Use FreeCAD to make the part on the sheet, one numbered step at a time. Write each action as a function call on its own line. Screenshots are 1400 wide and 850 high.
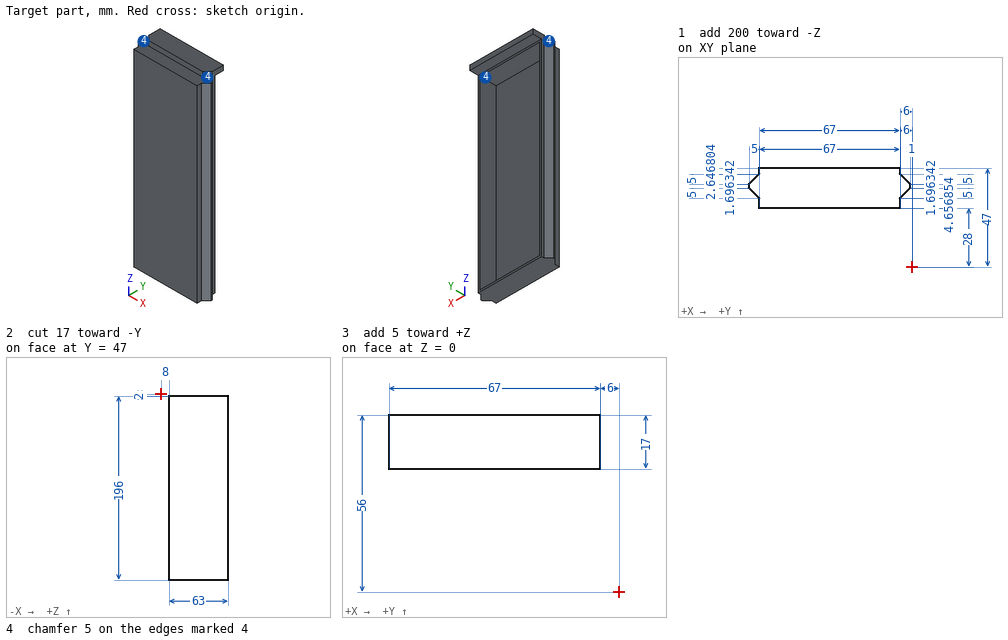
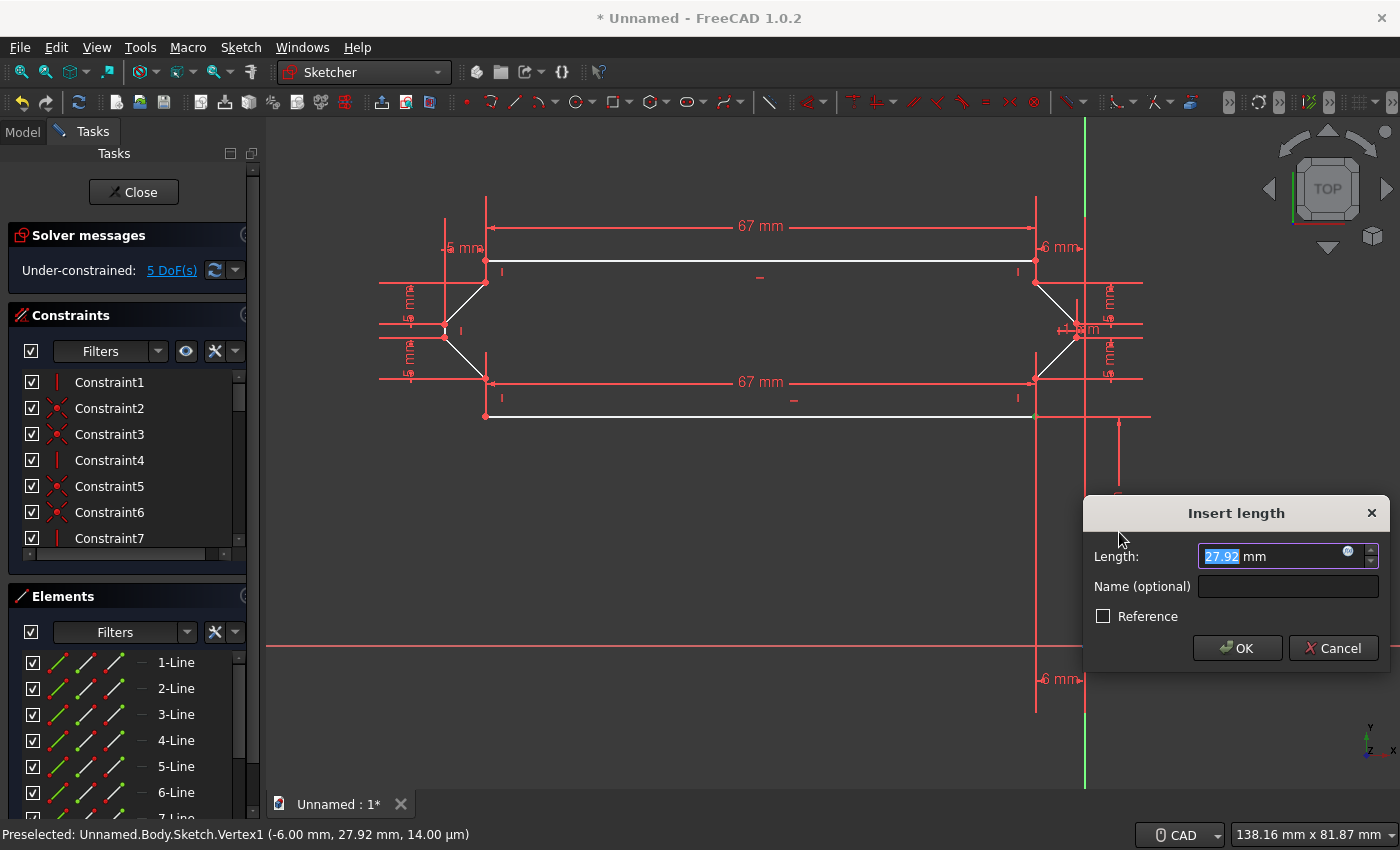
text(28)
key(Return)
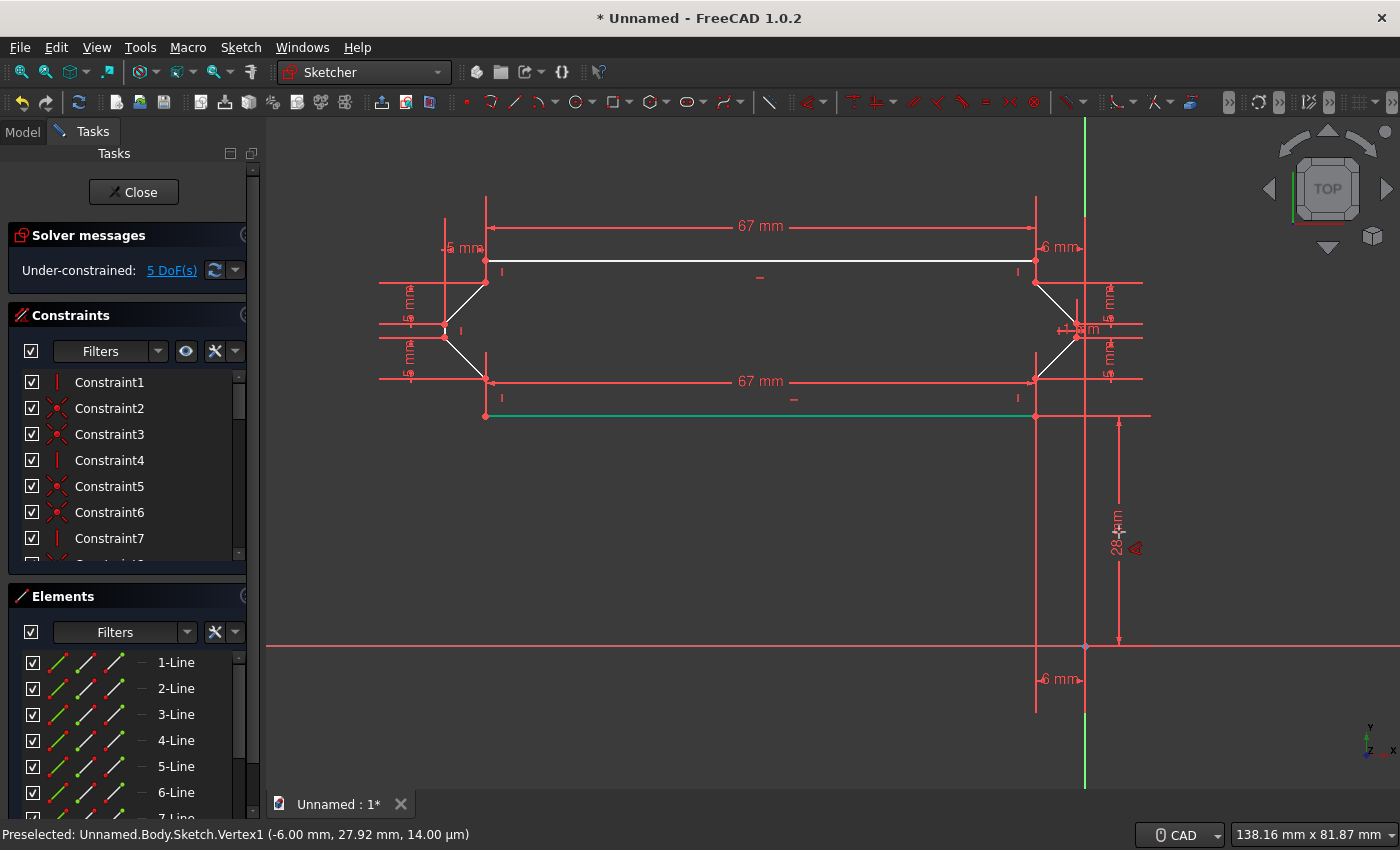
click(1036, 261)
click(1119, 454)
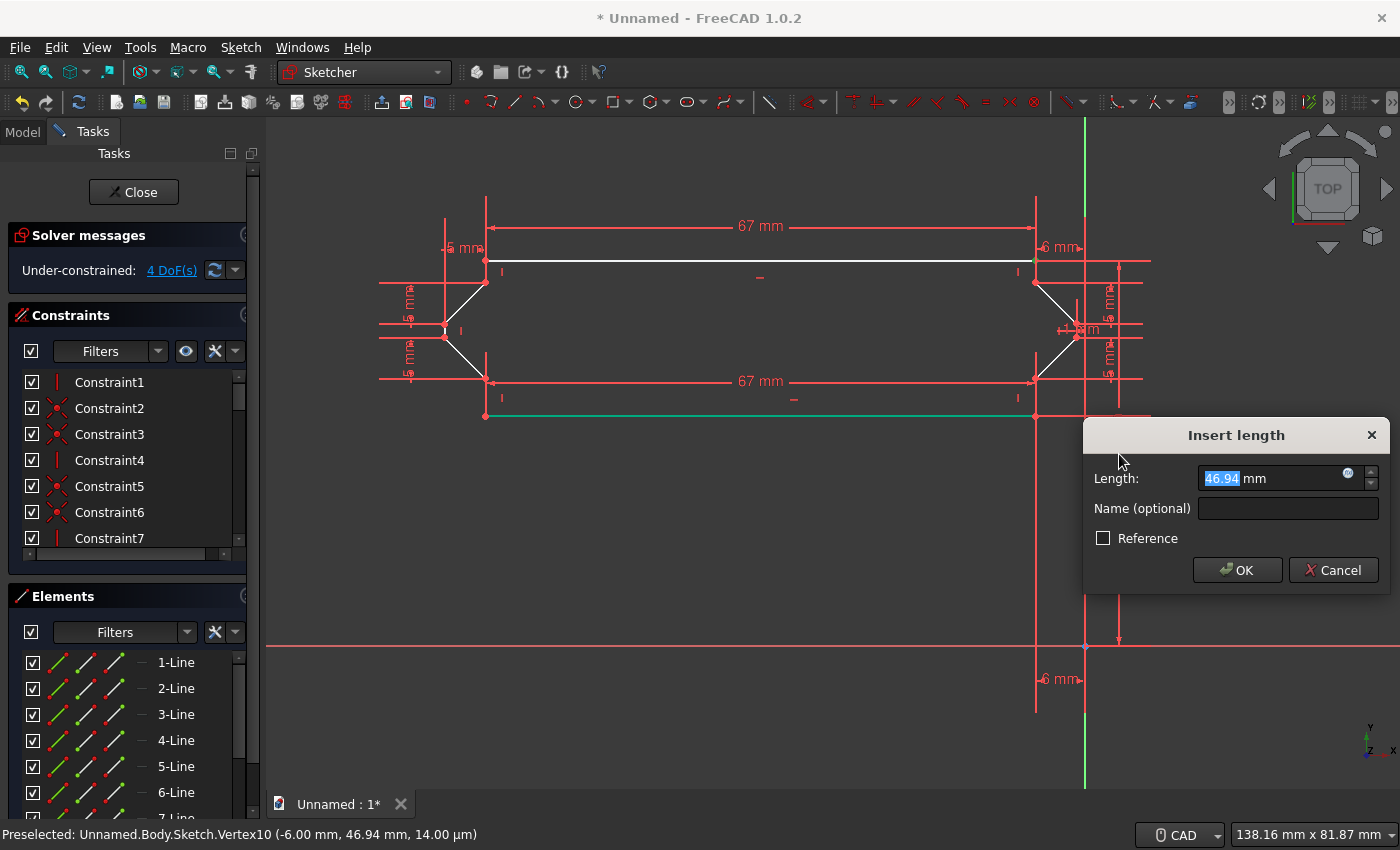
text(47)
key(Return)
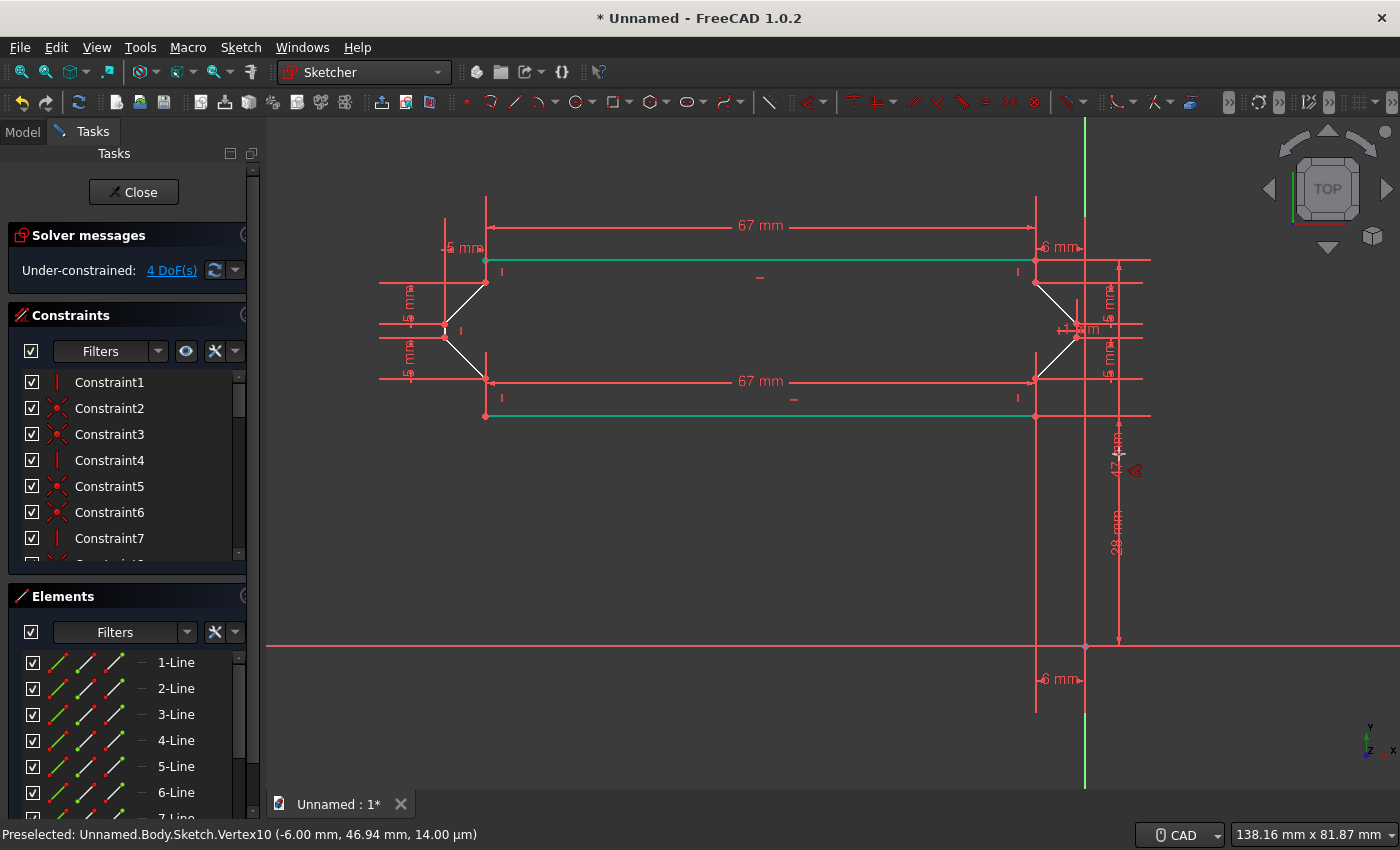
scroll(1036, 405, up, 2)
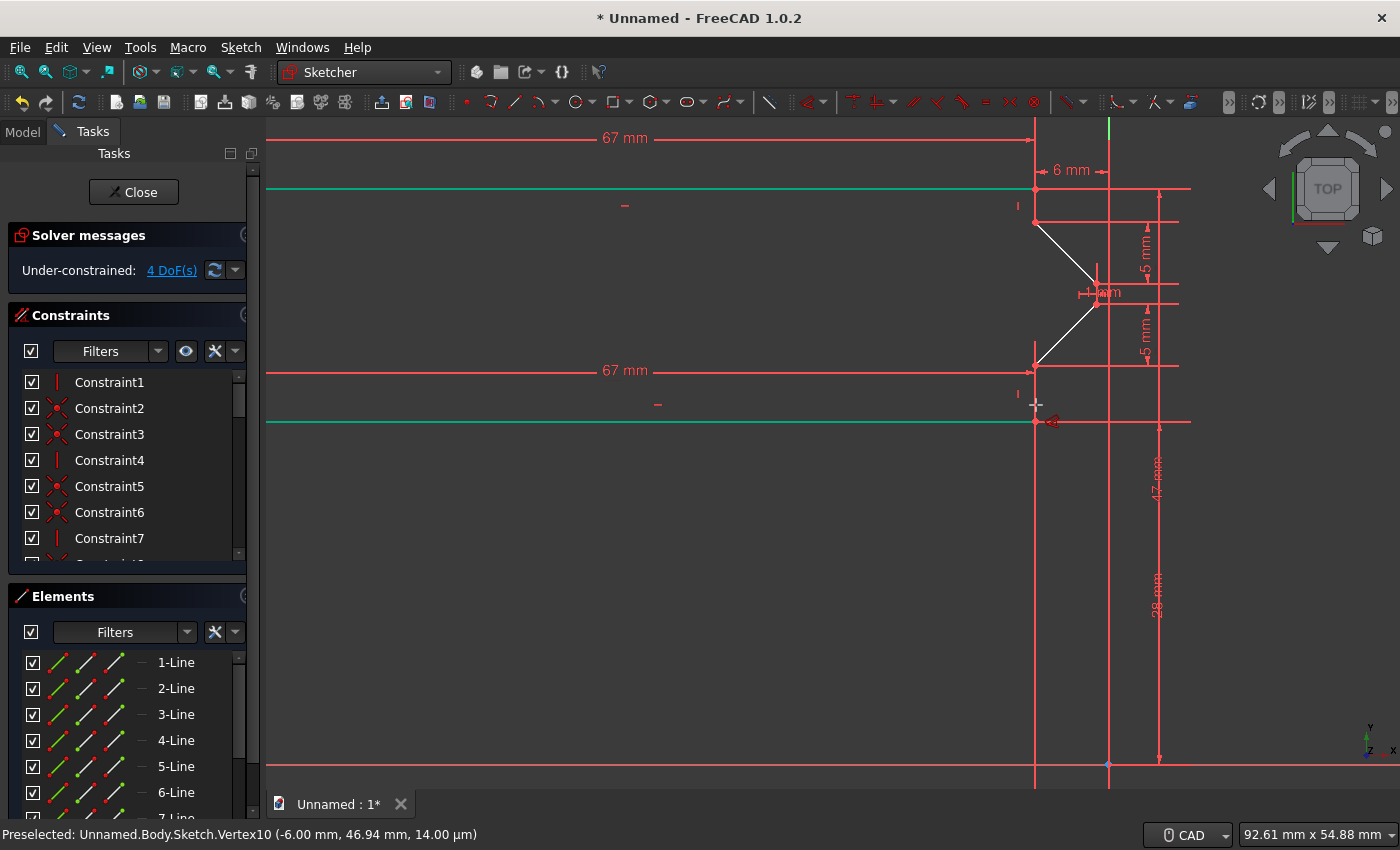
click(1035, 405)
click(1069, 394)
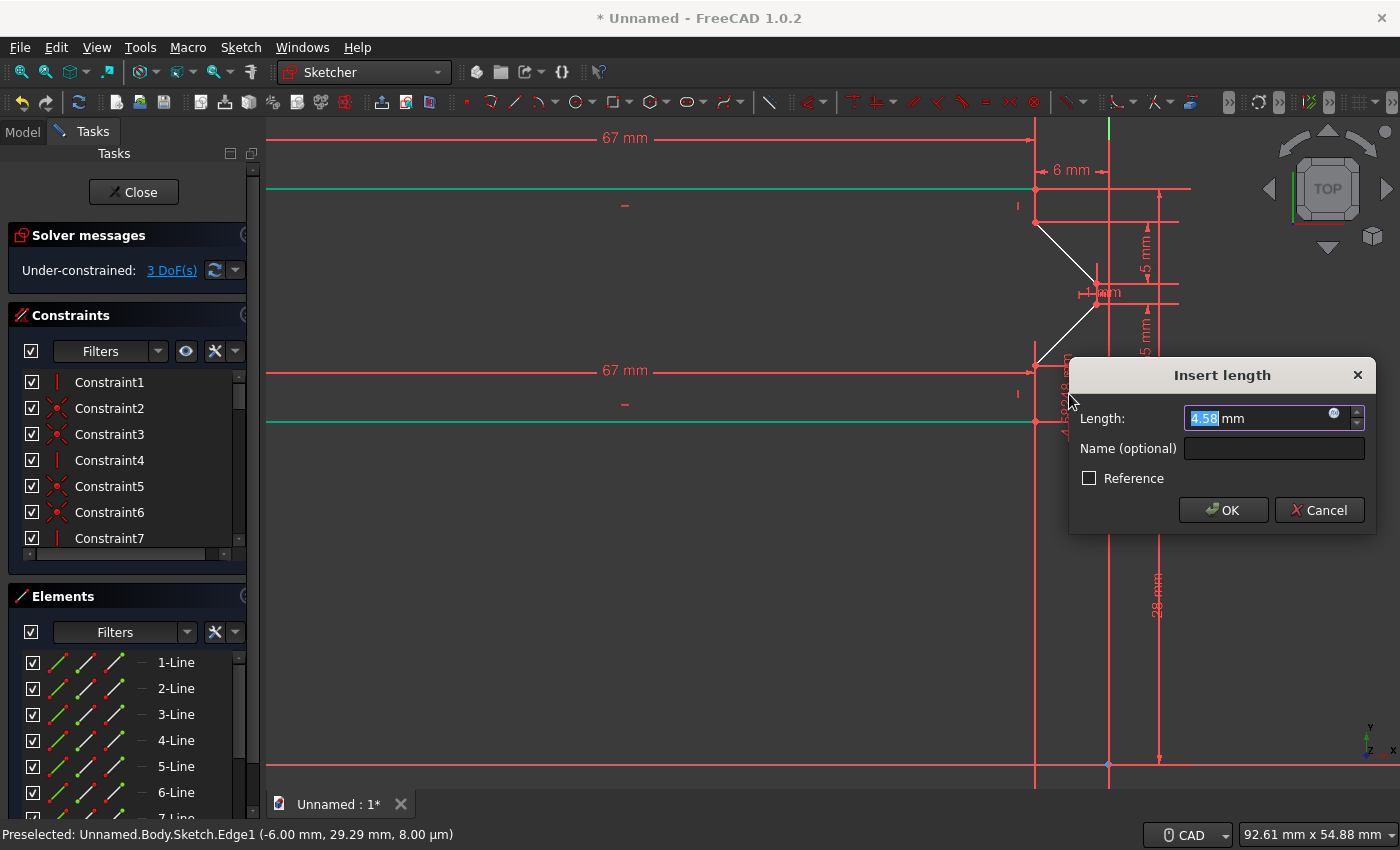
text(4.656854)
key(Return)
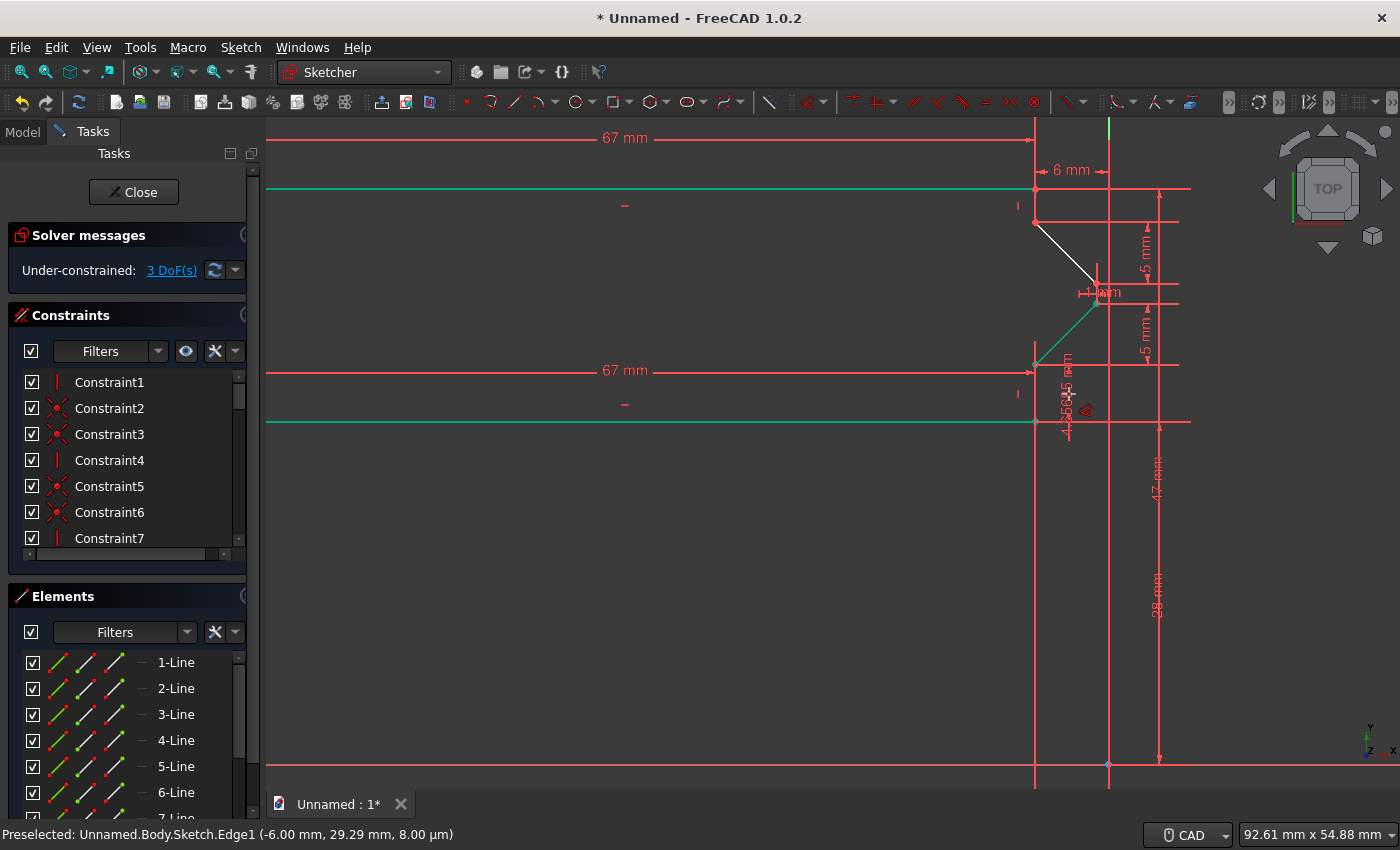
scroll(1097, 294, up, 4)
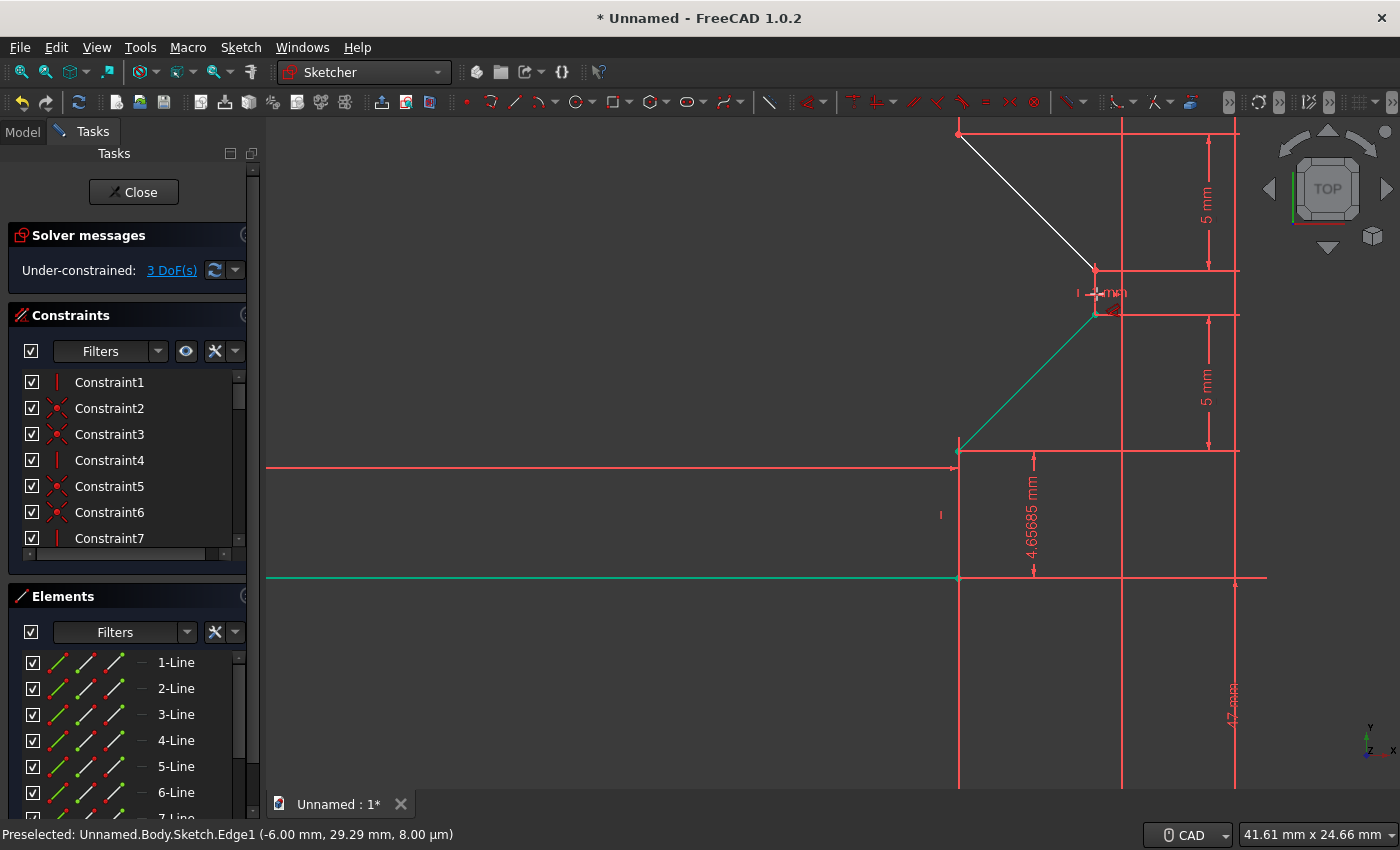
click(1095, 293)
click(1037, 293)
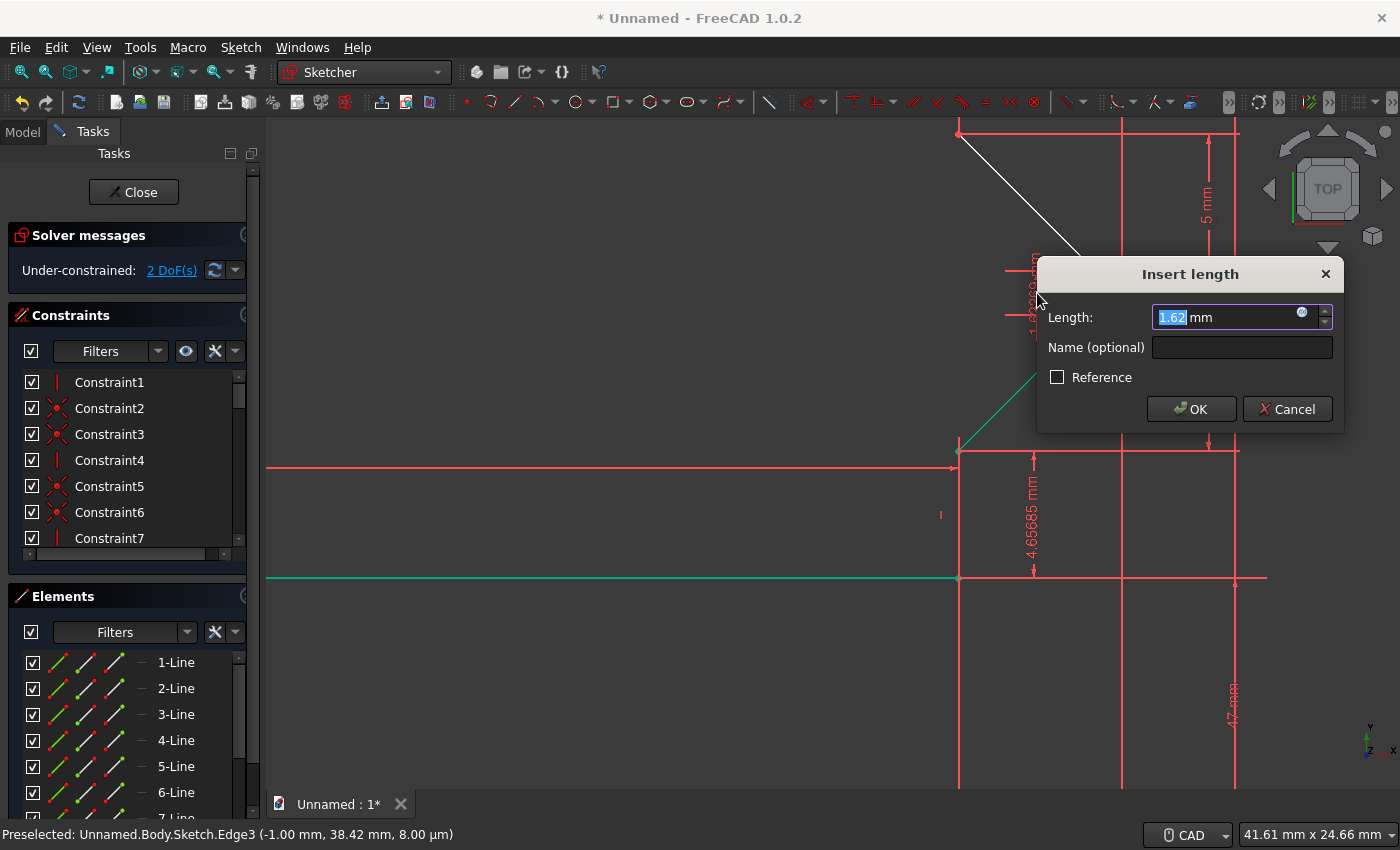
text(1.696342)
key(Return)